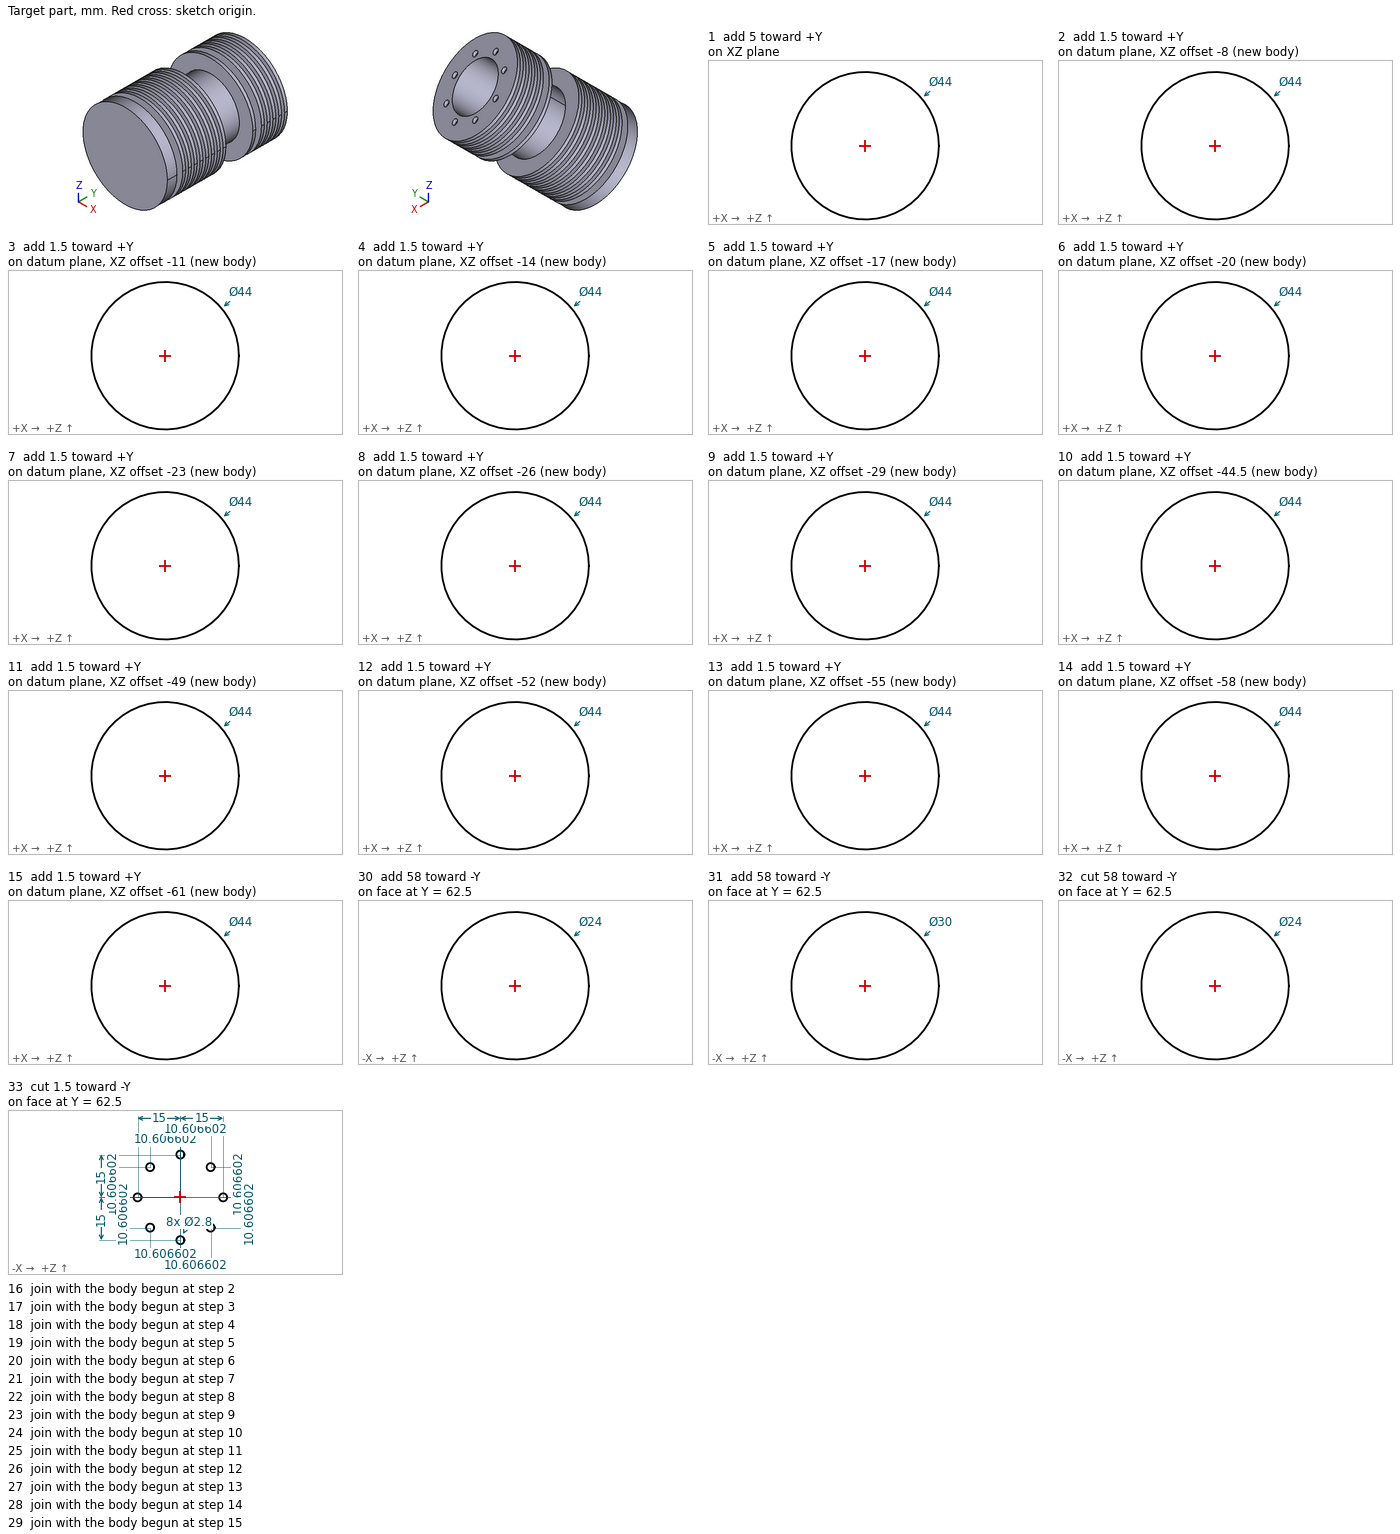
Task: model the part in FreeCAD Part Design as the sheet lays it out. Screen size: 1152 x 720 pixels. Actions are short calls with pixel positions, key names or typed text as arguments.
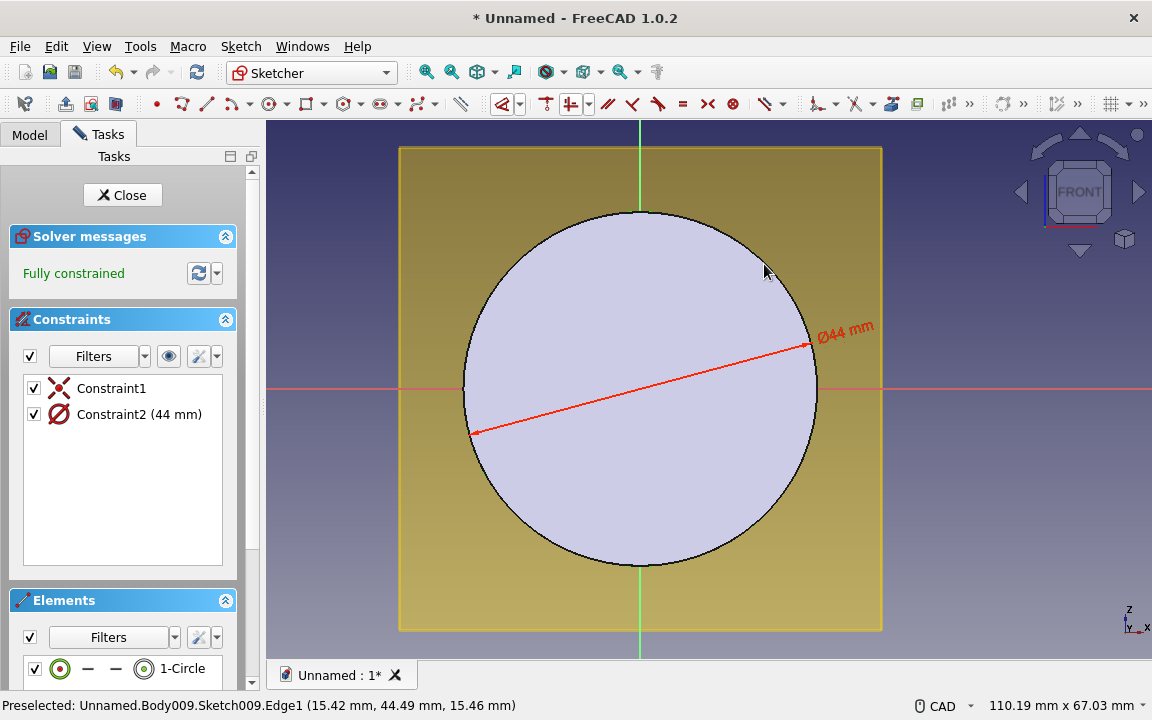
click(123, 195)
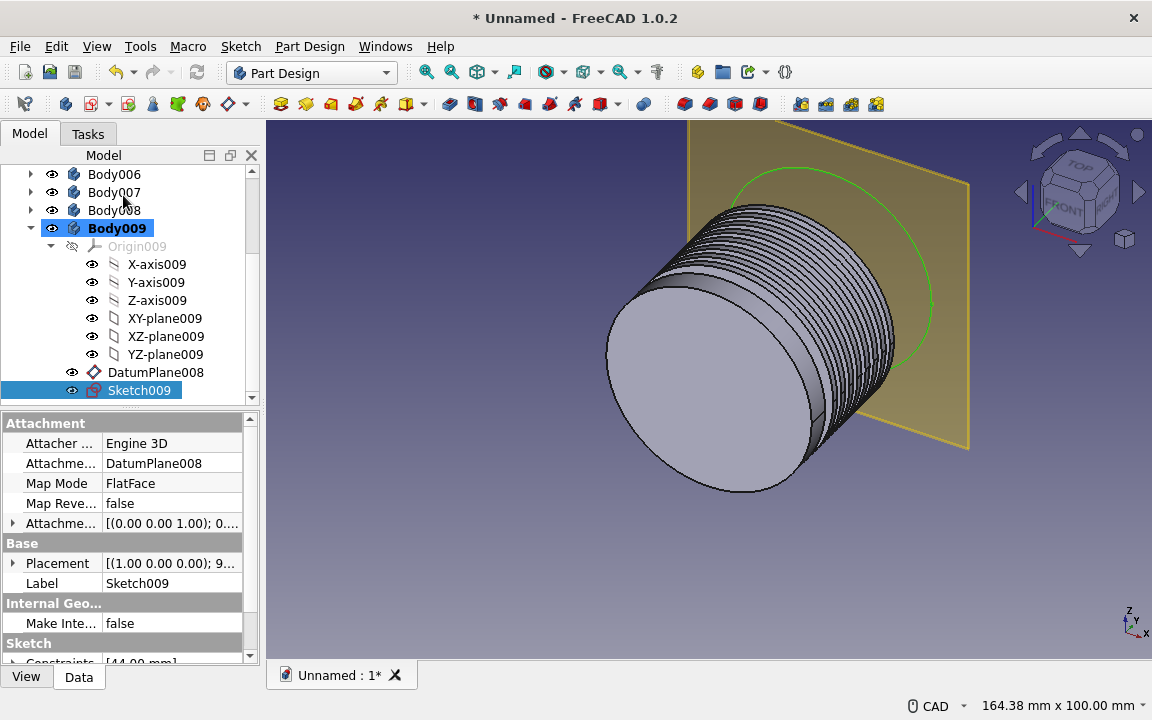
click(281, 104)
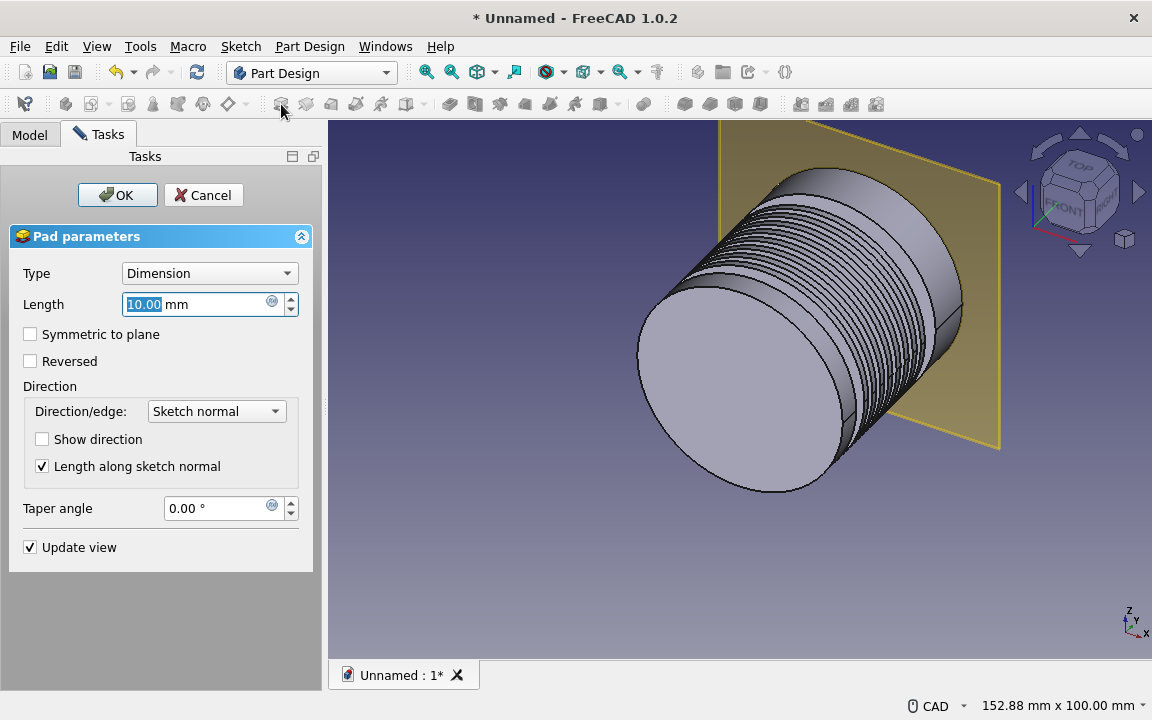
text(1.5)
key(Tab)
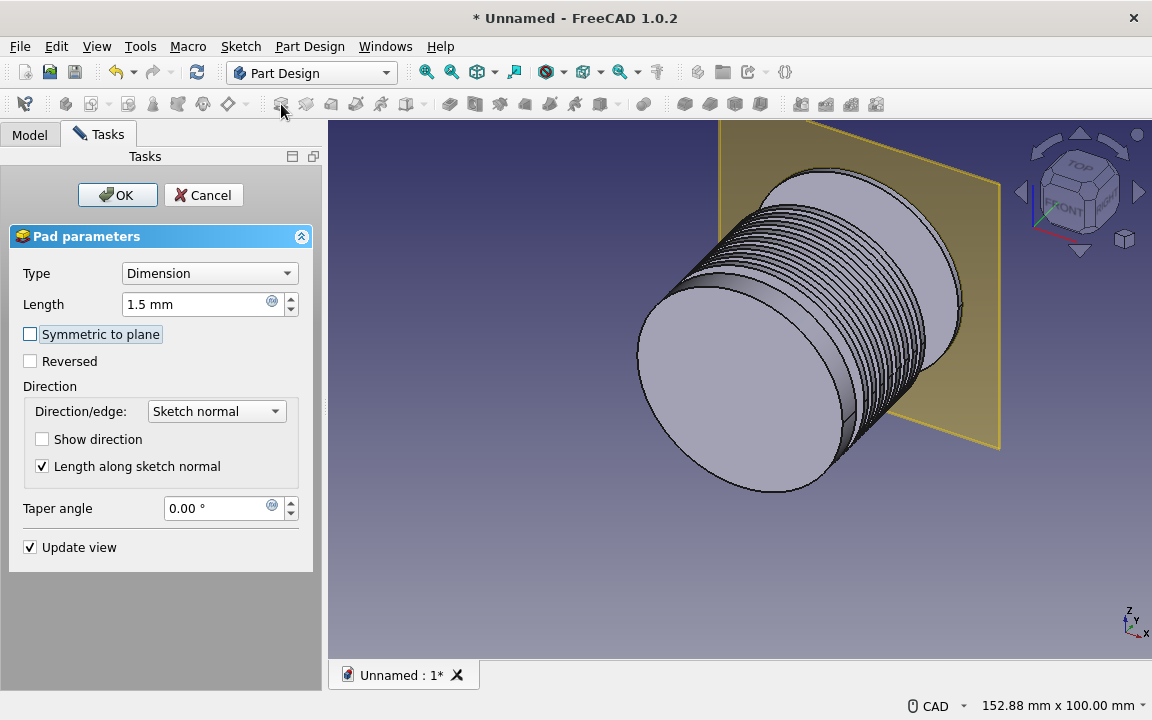
click(31, 361)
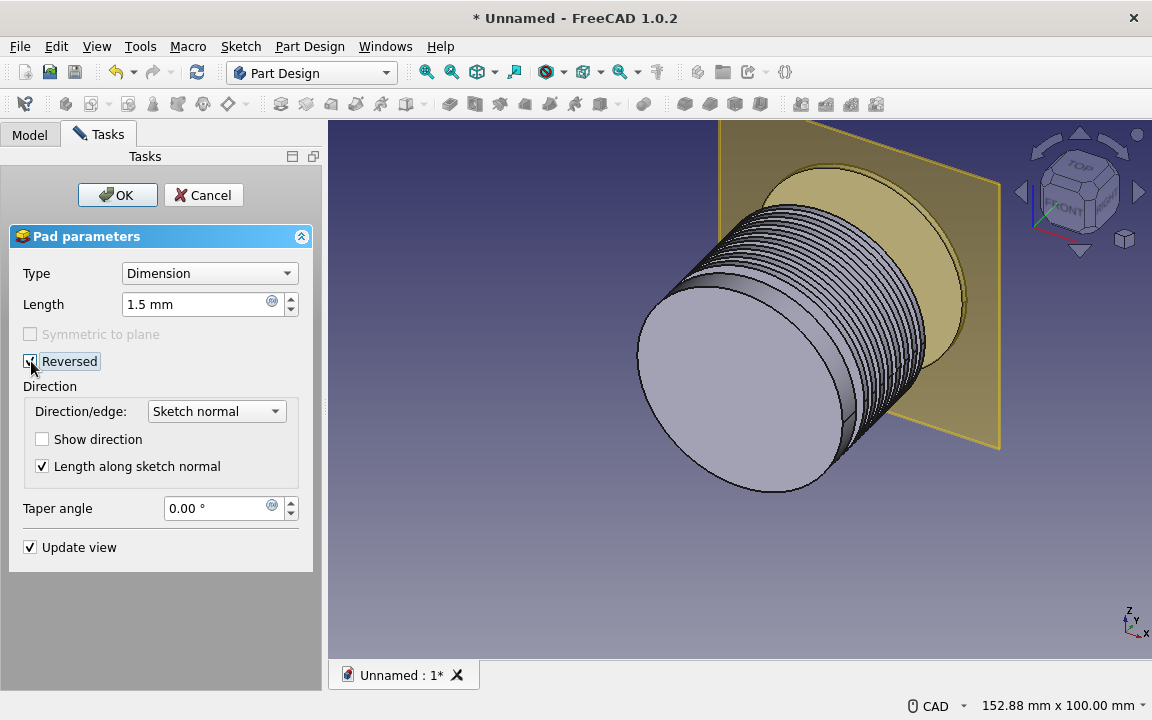
click(118, 195)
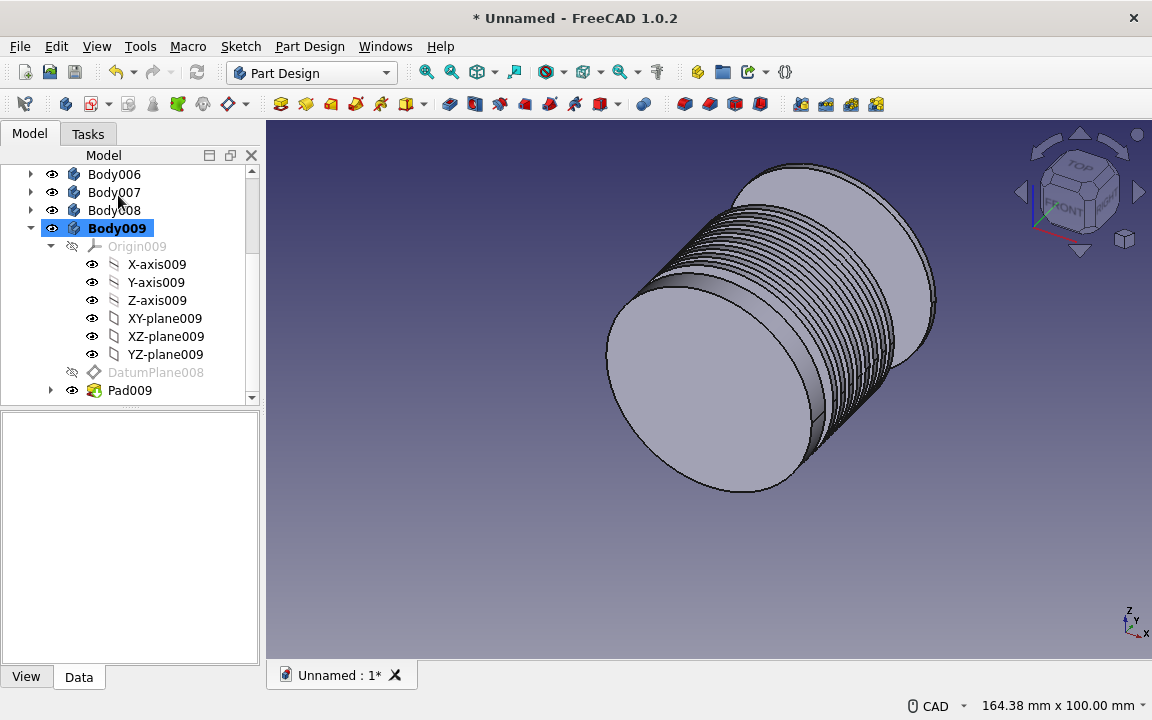
click(66, 104)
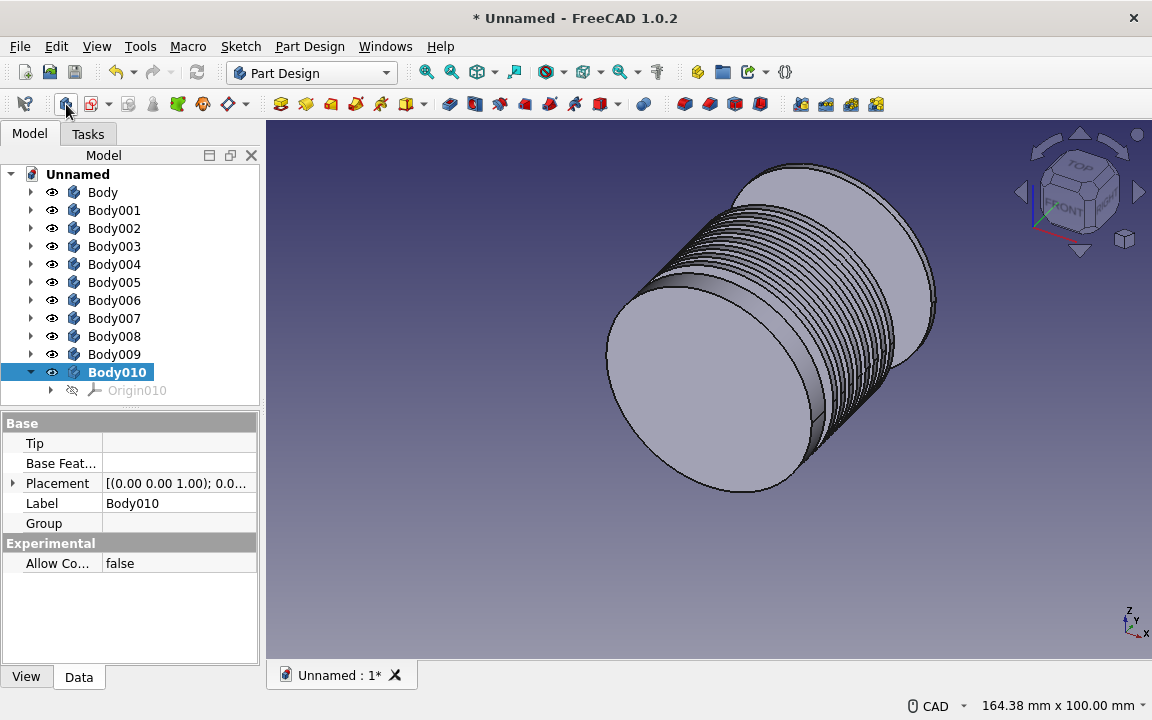
click(51, 390)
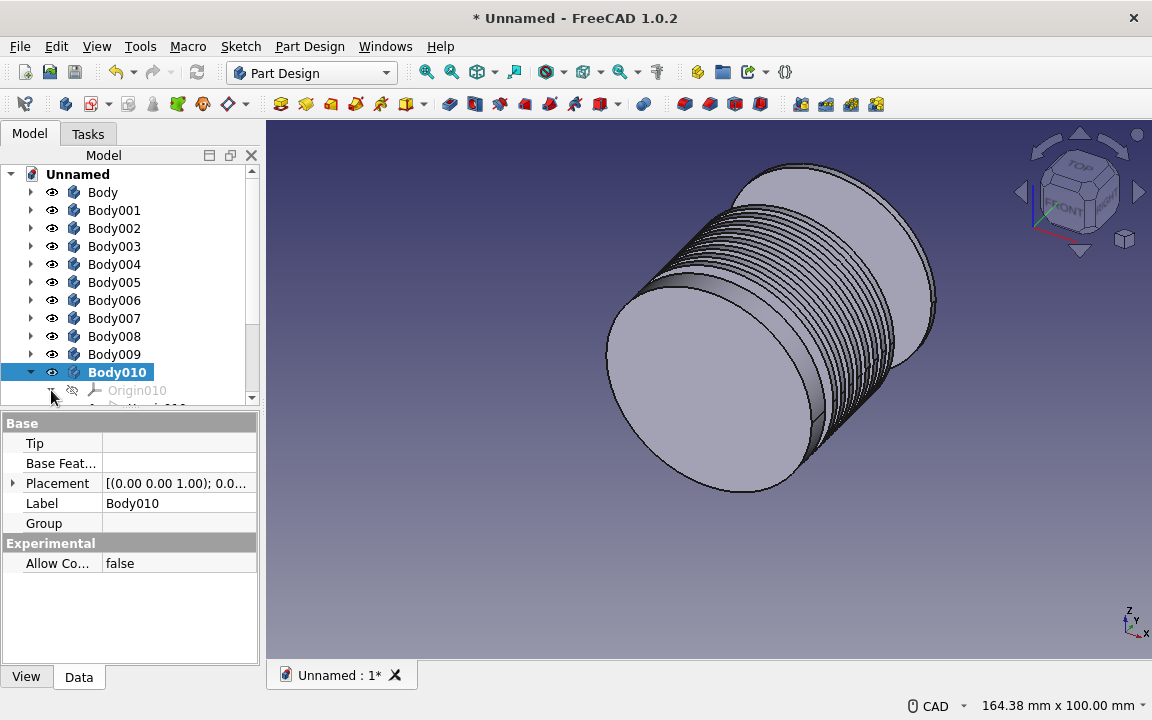
scroll(101, 278, down, 3)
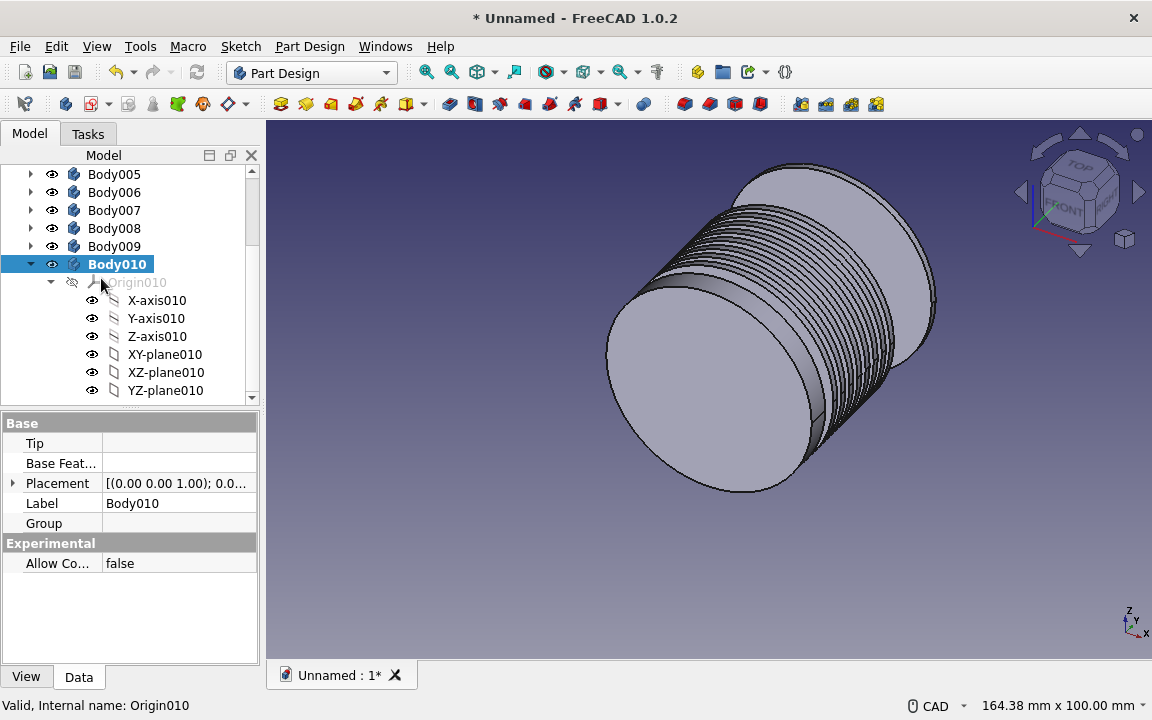
click(137, 372)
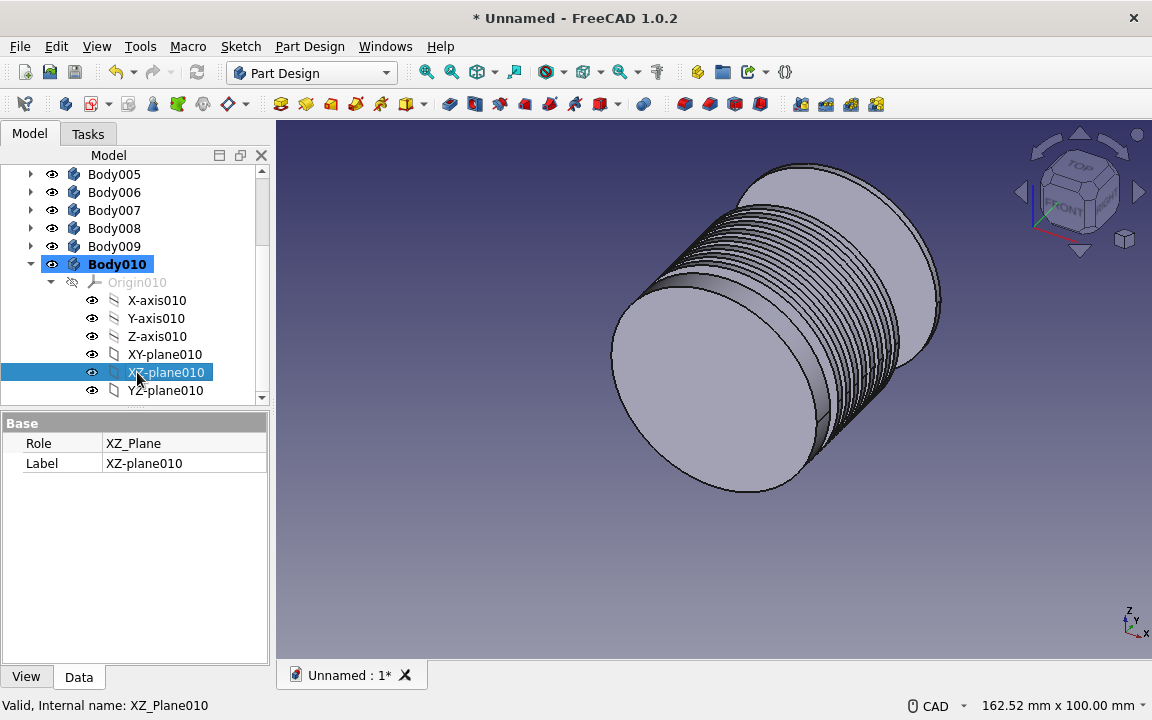
click(228, 104)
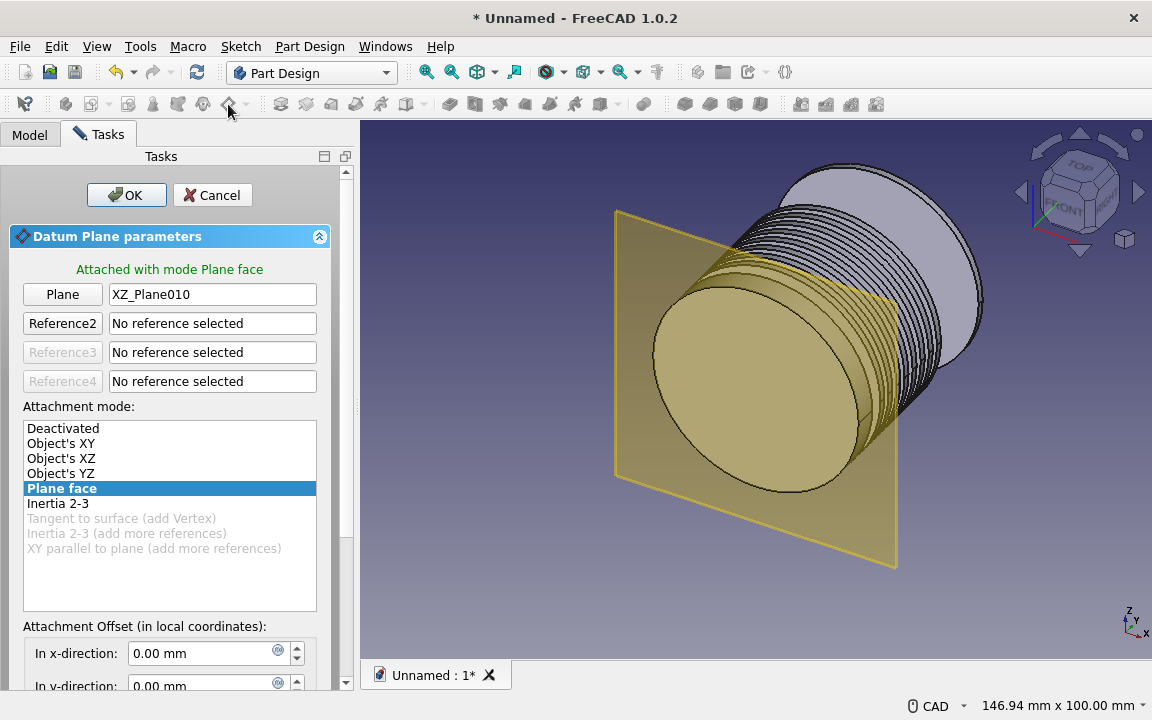
scroll(346, 428, down, 2)